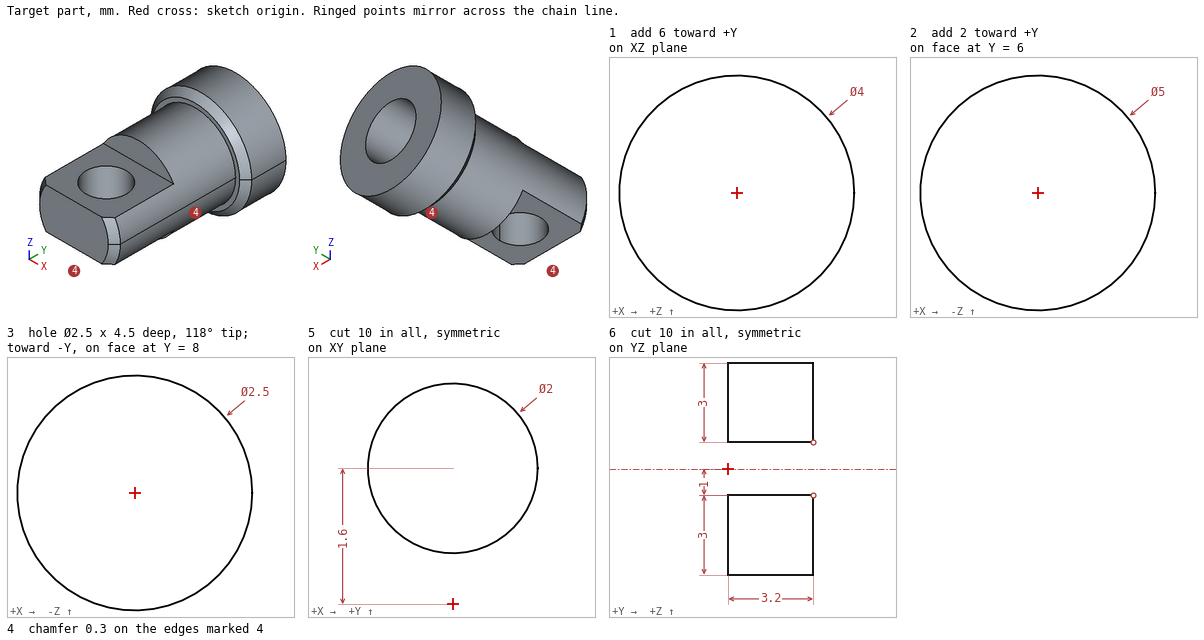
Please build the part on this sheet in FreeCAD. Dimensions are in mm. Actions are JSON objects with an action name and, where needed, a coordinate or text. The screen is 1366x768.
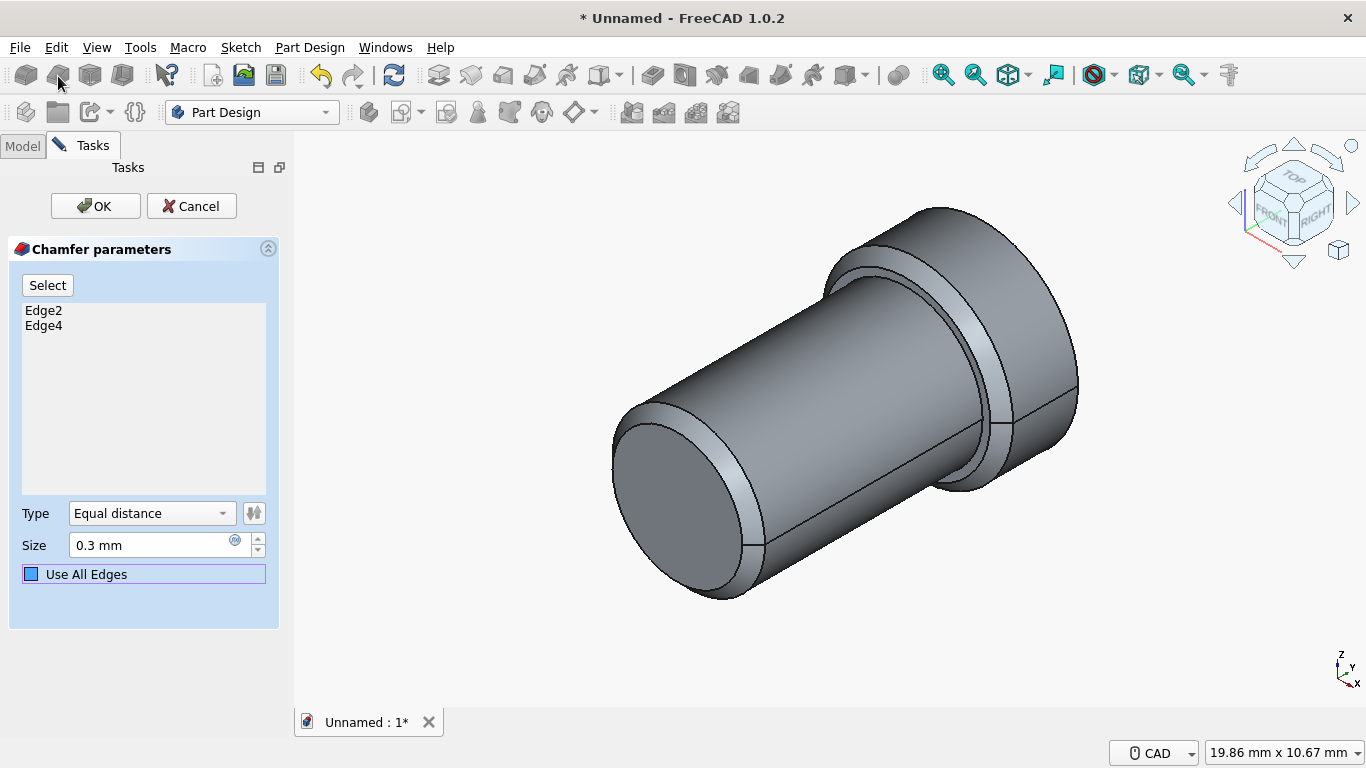
{"action": "left_click", "coordinate": [96, 206]}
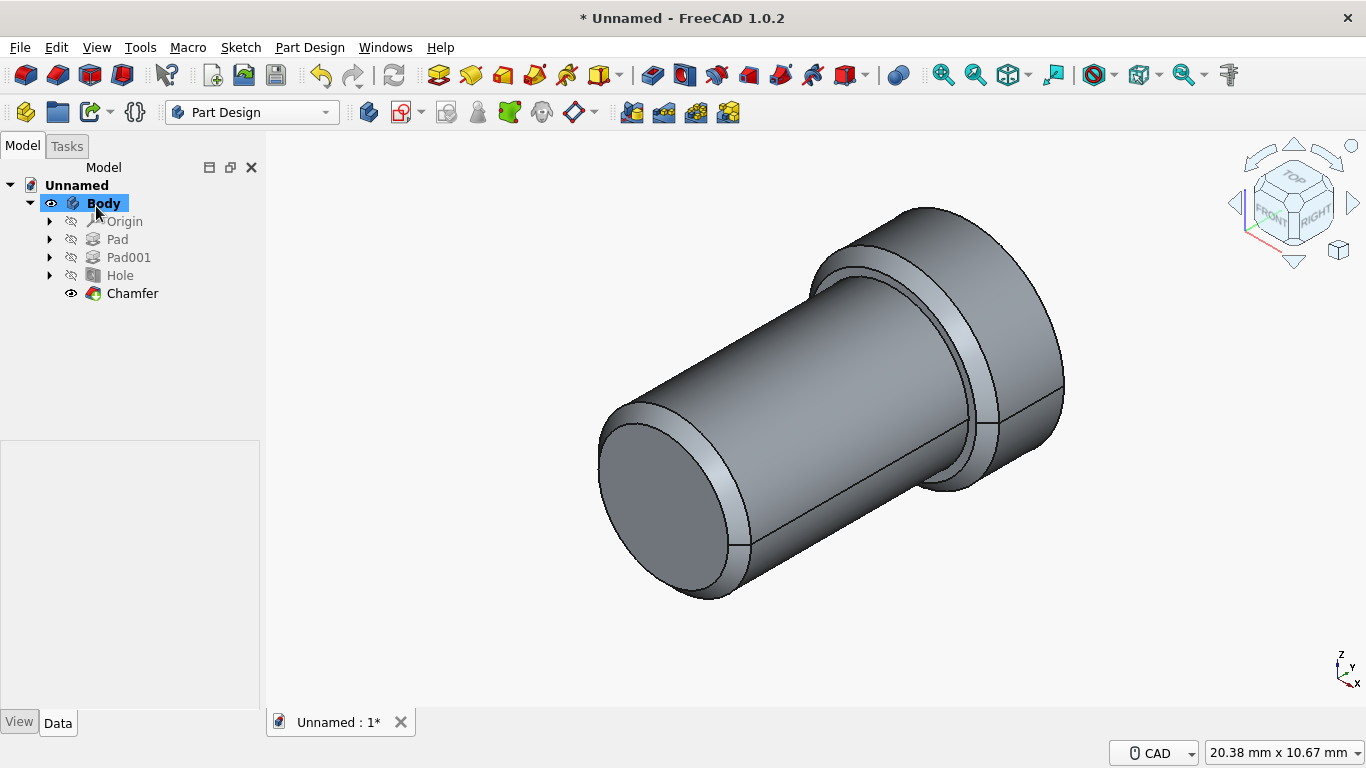
{"action": "left_click", "coordinate": [402, 112]}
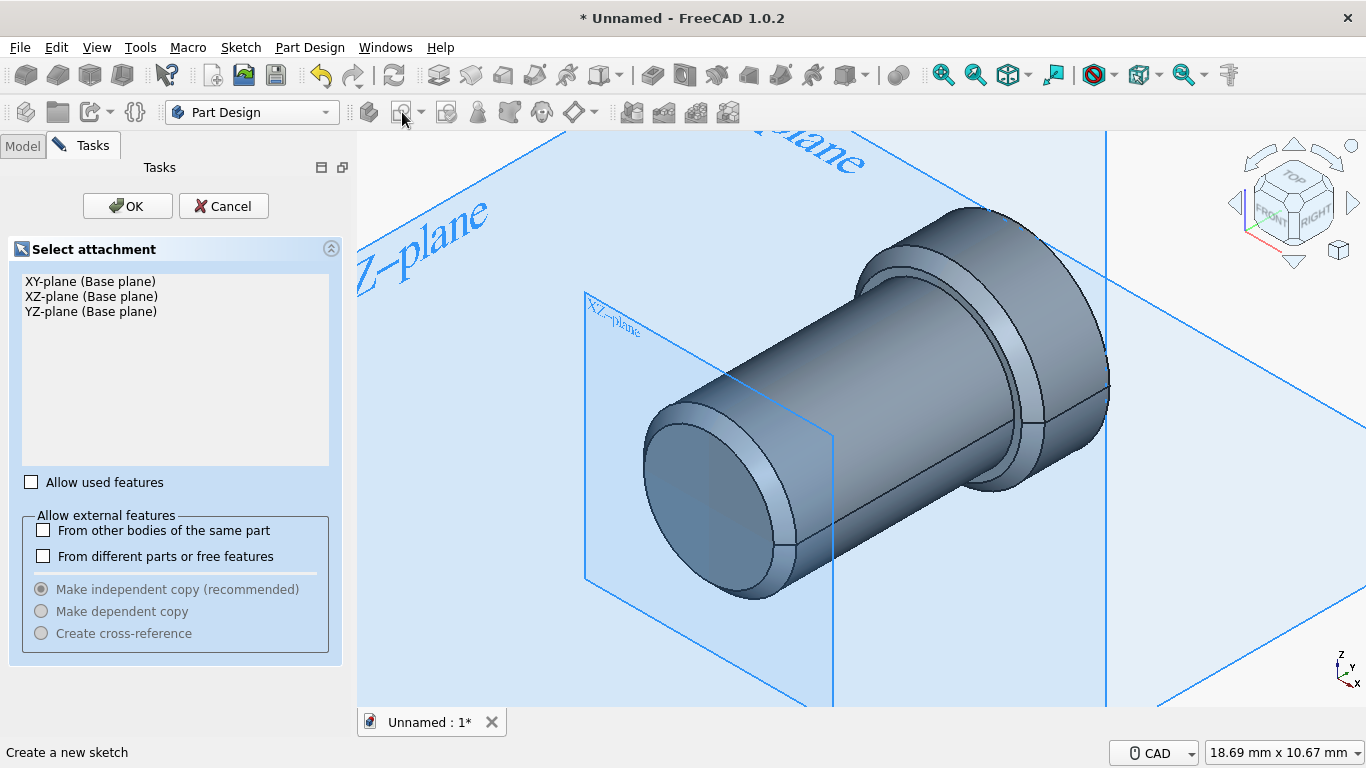
{"action": "left_click", "coordinate": [82, 282]}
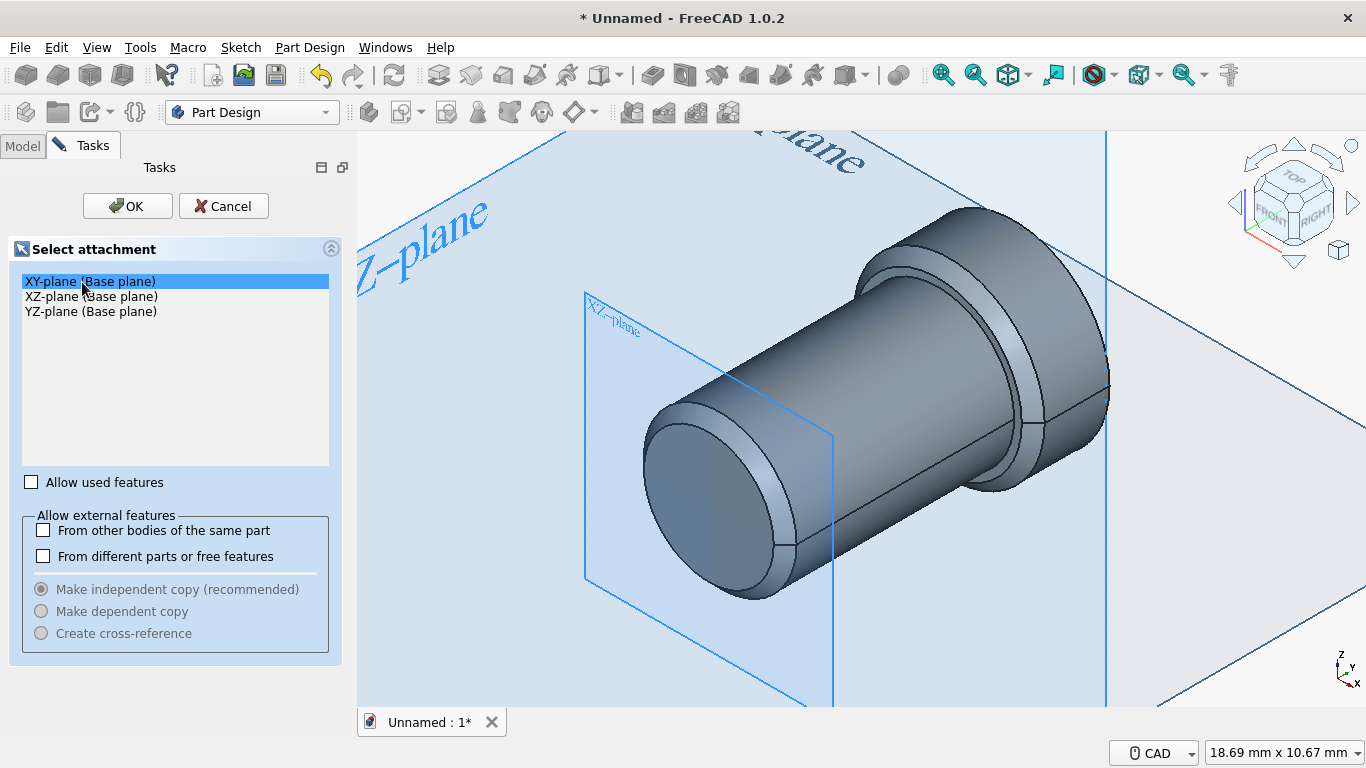
{"action": "left_click", "coordinate": [128, 206]}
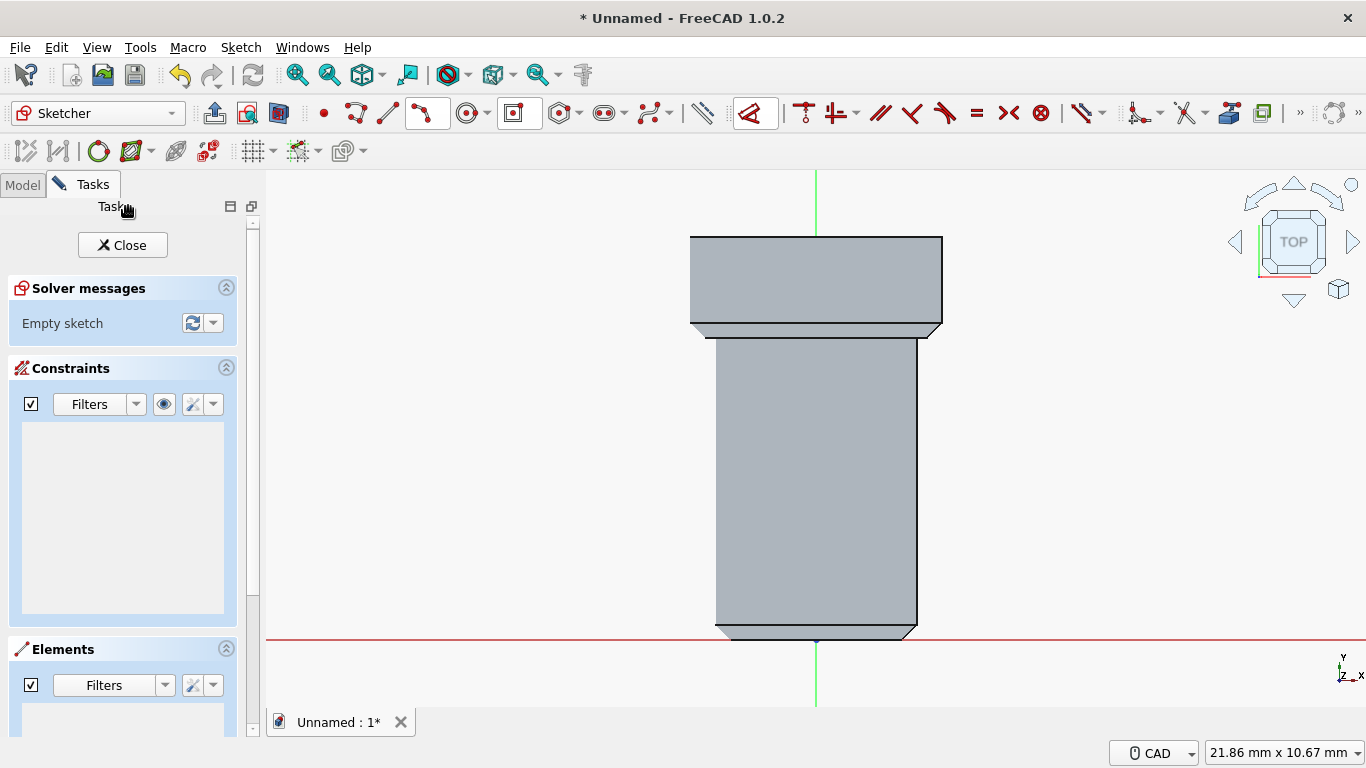
{"action": "key", "text": "q s"}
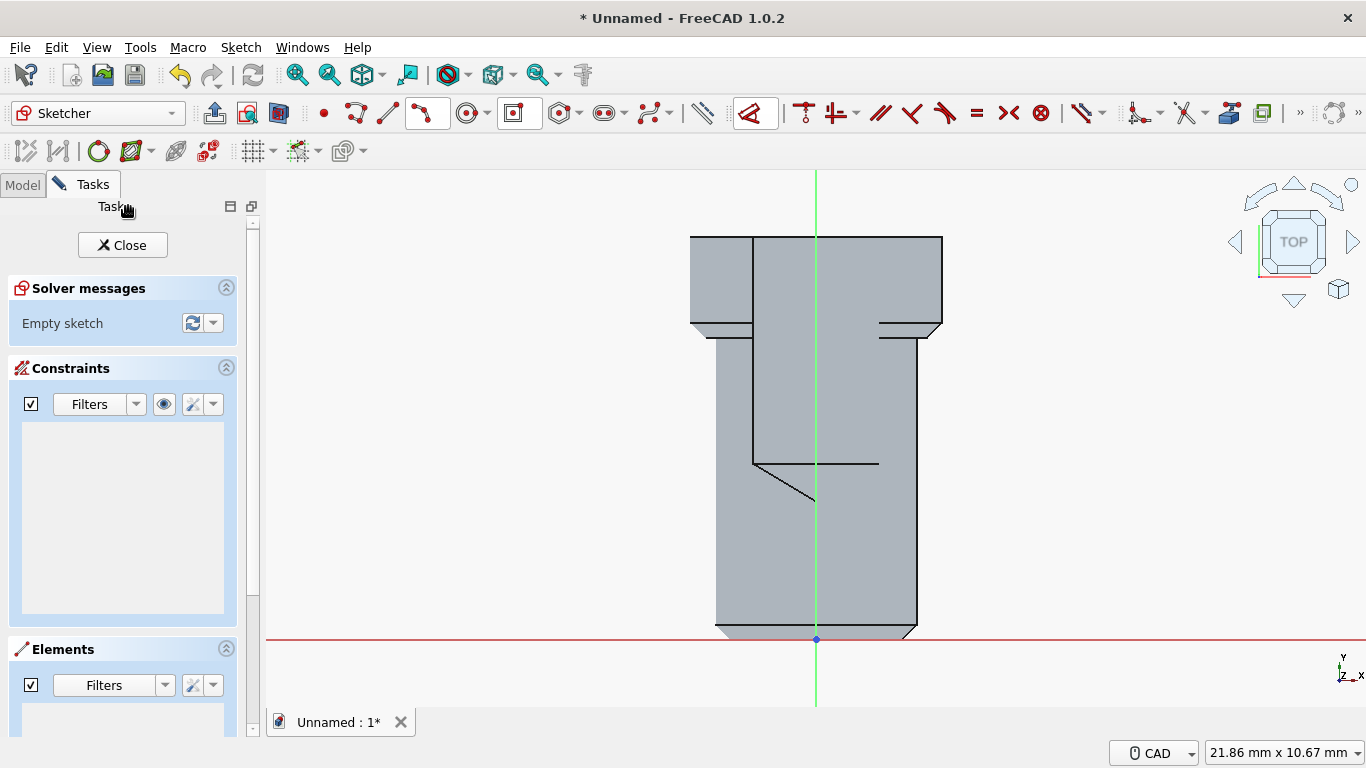
{"action": "scroll", "coordinate": [856, 653], "scroll_direction": "up", "scroll_amount": 5}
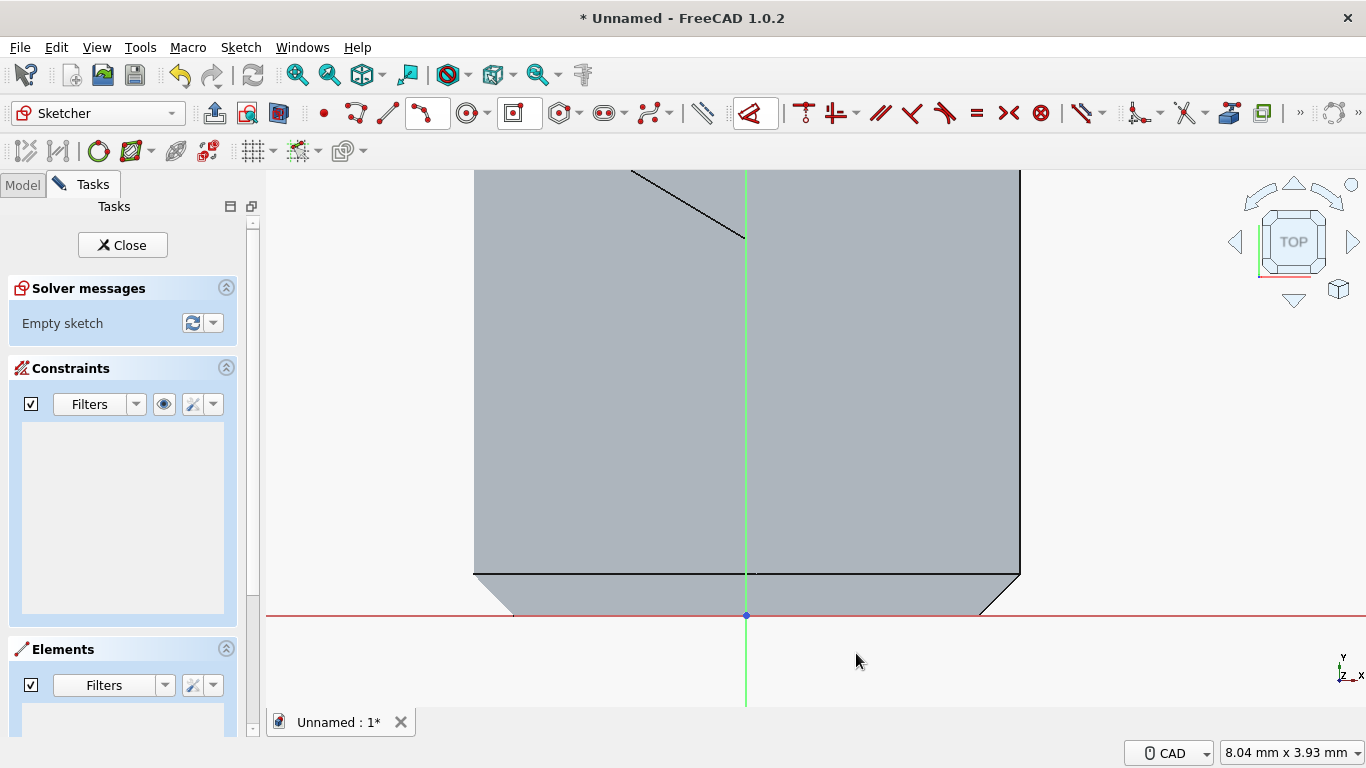
{"action": "left_click", "coordinate": [468, 114]}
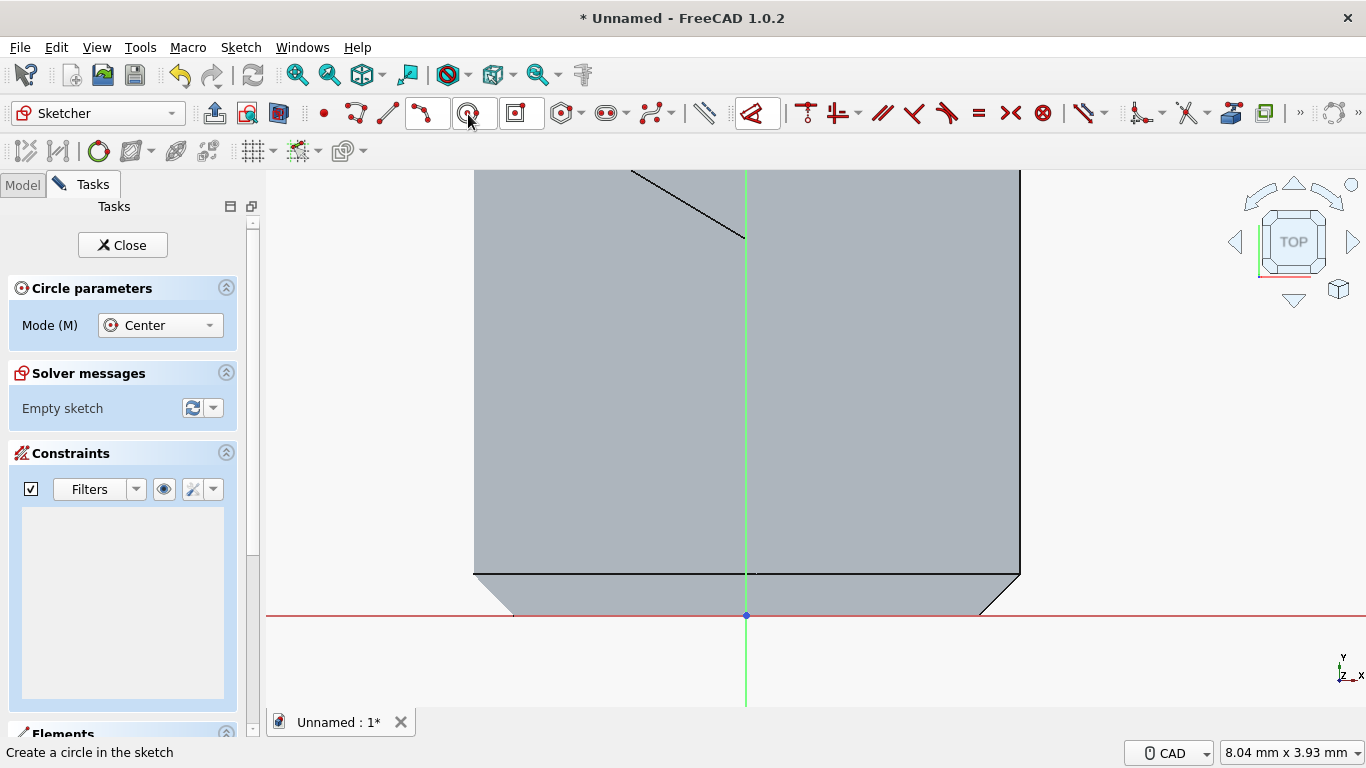
{"action": "left_click", "coordinate": [746, 397]}
{"action": "left_click", "coordinate": [843, 300]}
{"action": "key", "text": "Escape"}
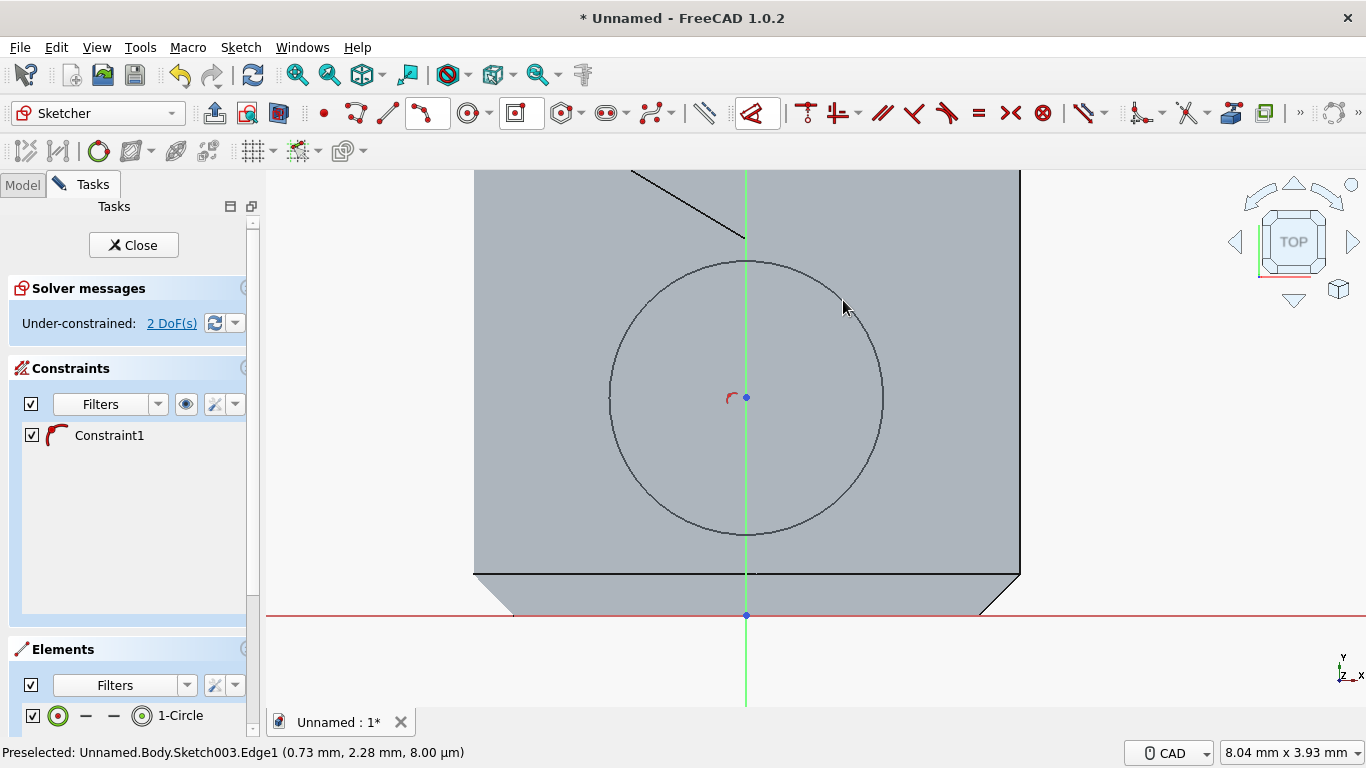
{"action": "left_click", "coordinate": [843, 301]}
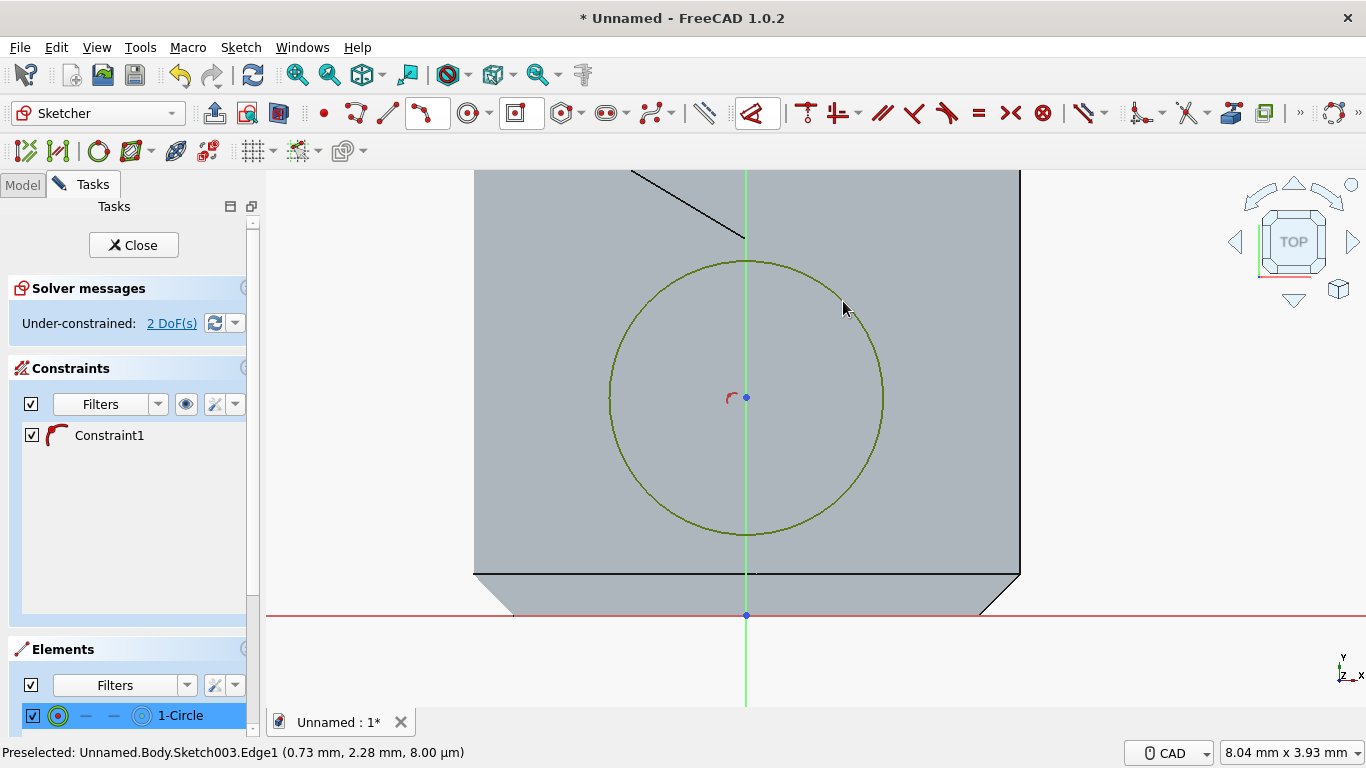
{"action": "key", "text": "k o"}